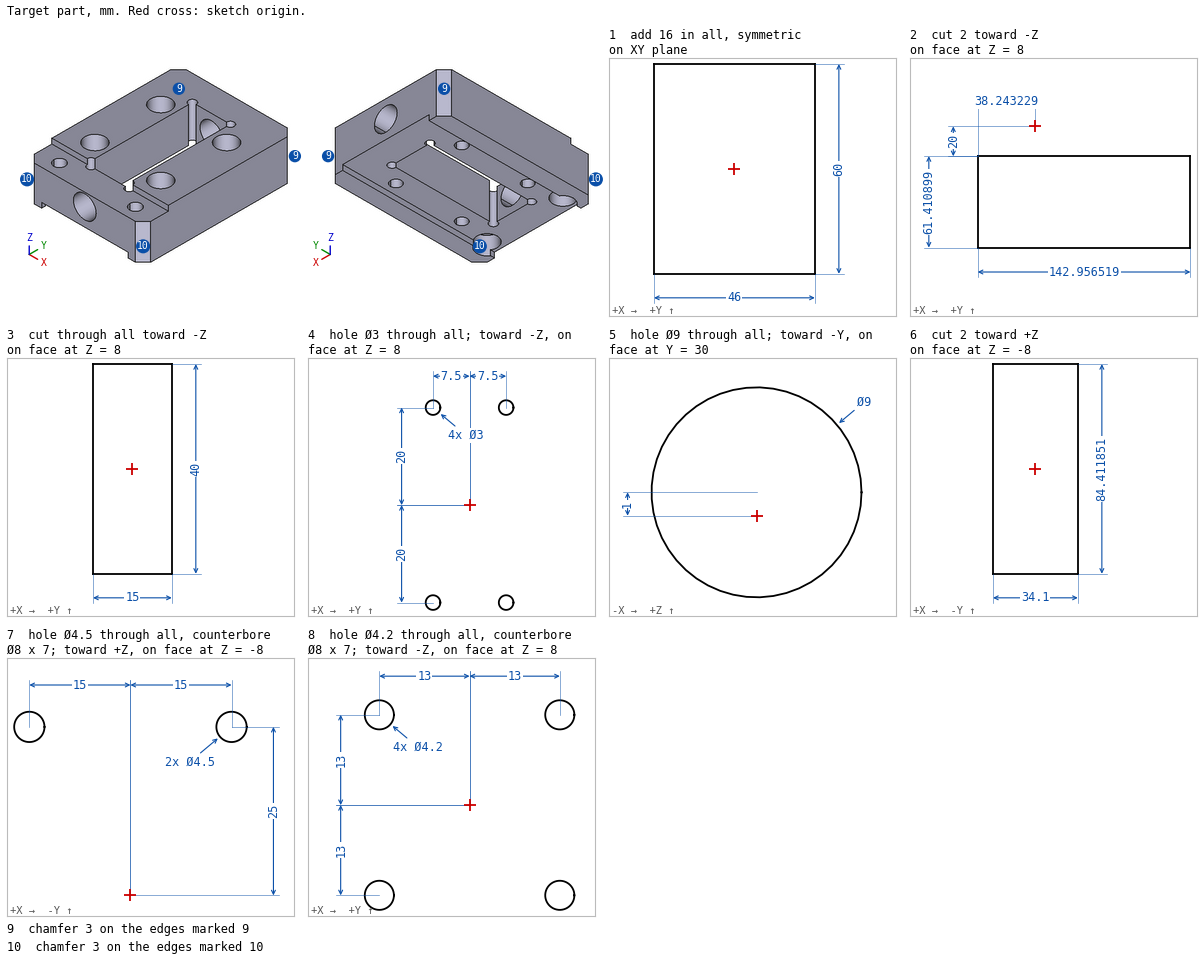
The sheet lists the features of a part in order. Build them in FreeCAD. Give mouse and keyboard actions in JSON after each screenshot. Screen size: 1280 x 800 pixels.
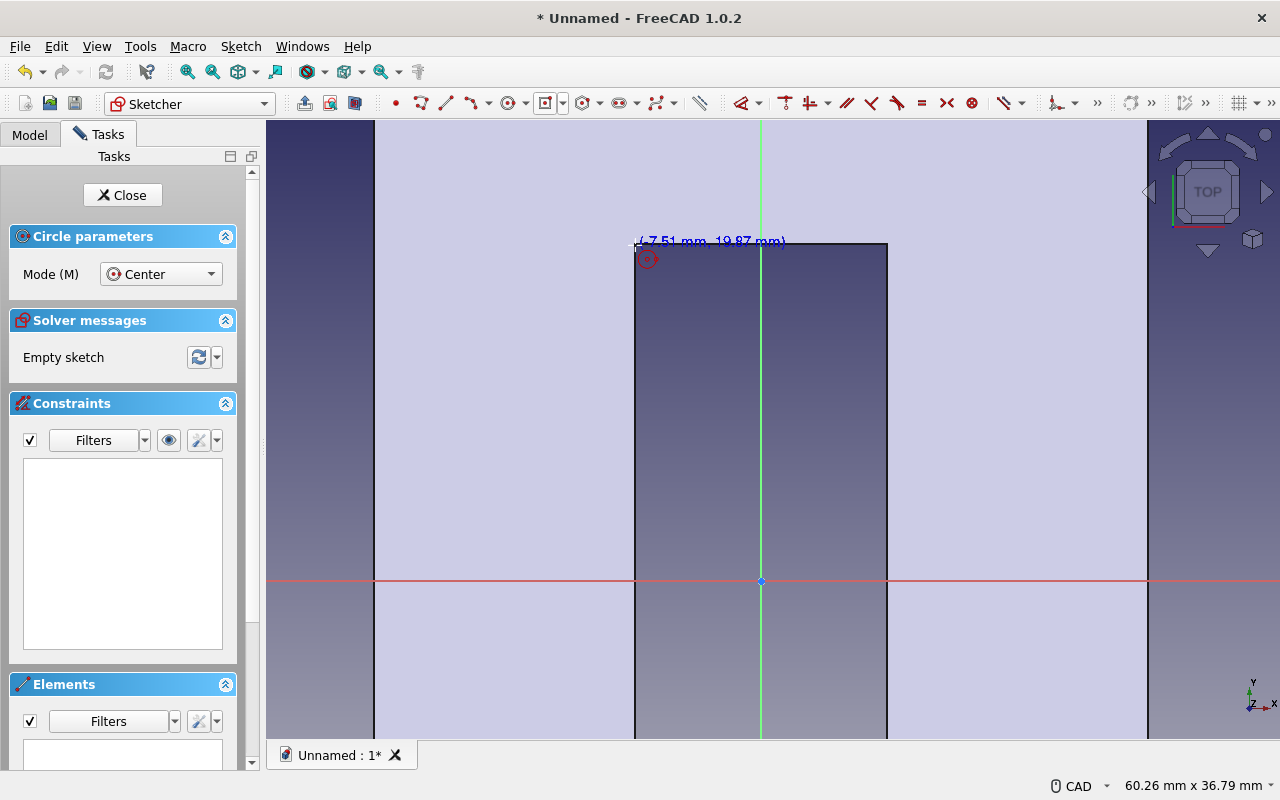
{"action": "left_click", "coordinate": [635, 244]}
{"action": "left_click", "coordinate": [653, 227]}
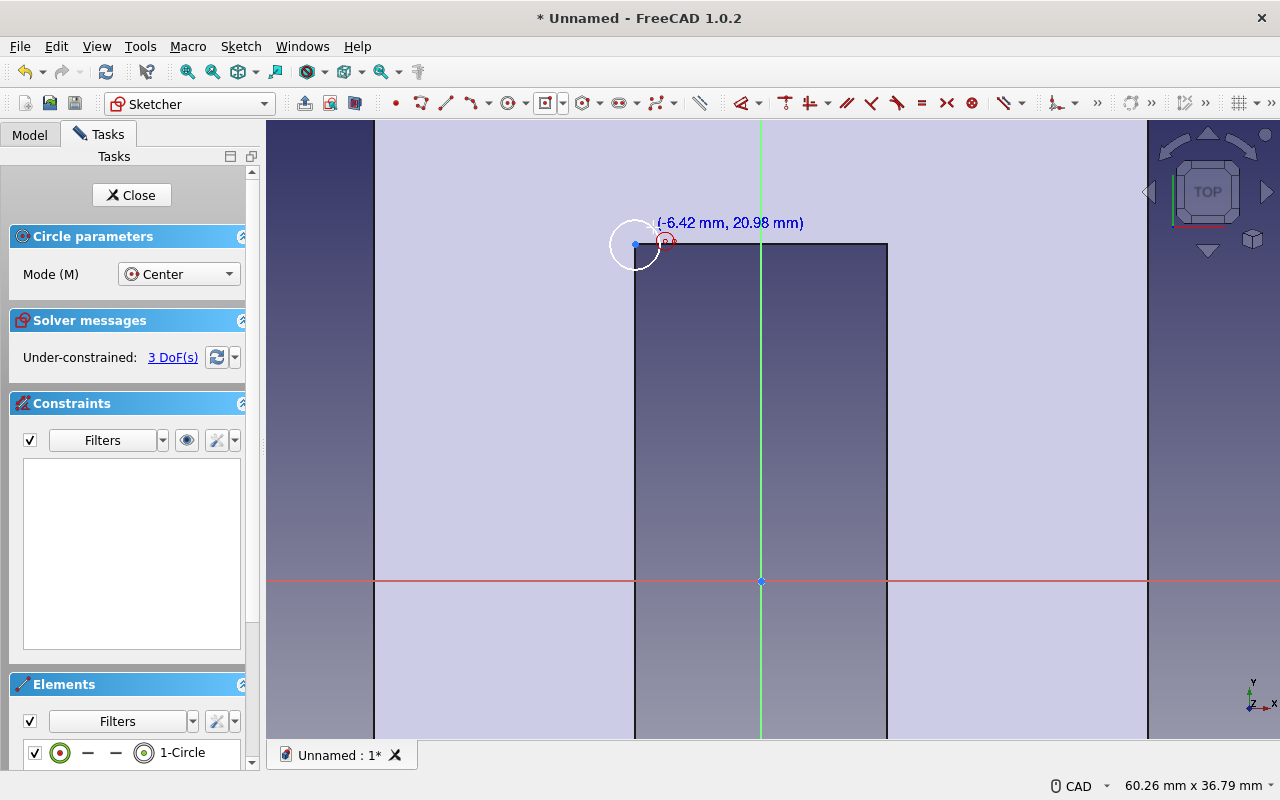
{"action": "left_click", "coordinate": [887, 244]}
{"action": "left_click", "coordinate": [905, 227]}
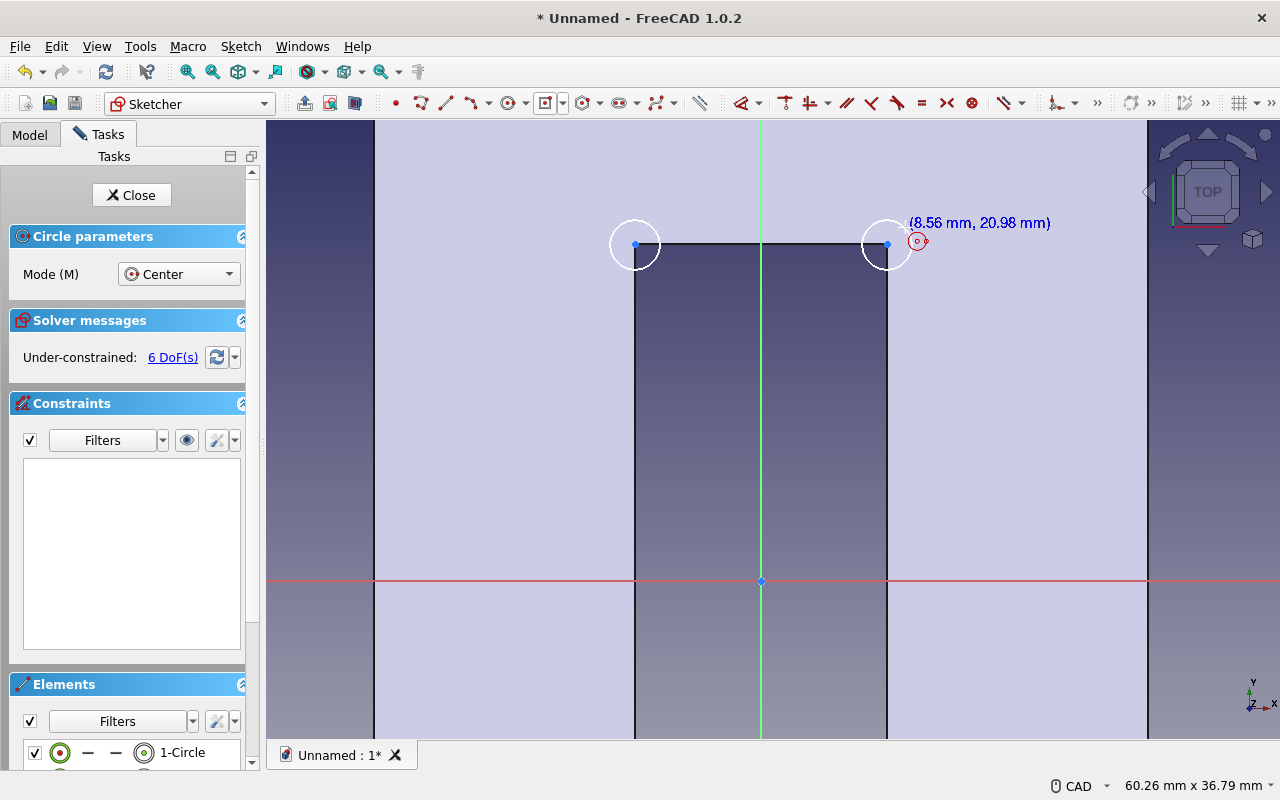
{"action": "scroll", "coordinate": [636, 245], "scroll_direction": "down", "scroll_amount": 3}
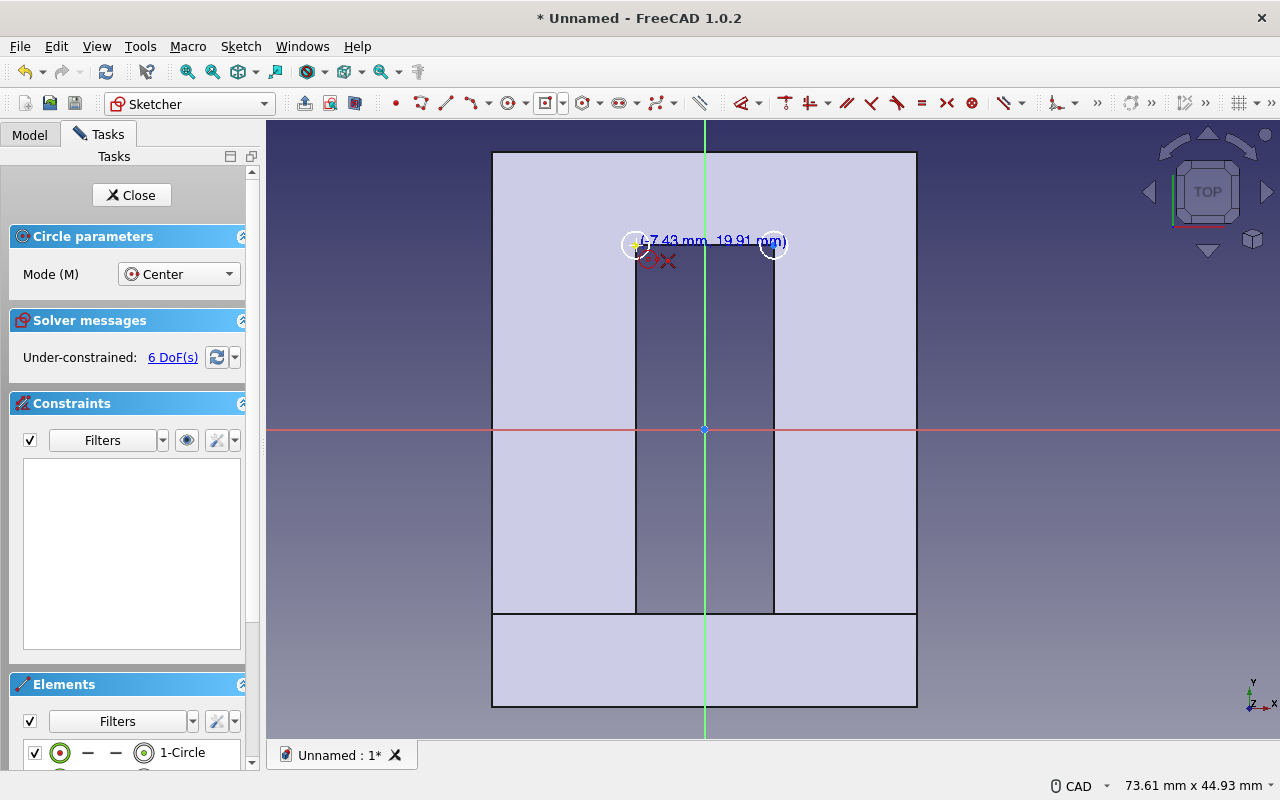
{"action": "scroll", "coordinate": [636, 614], "scroll_direction": "up", "scroll_amount": 3}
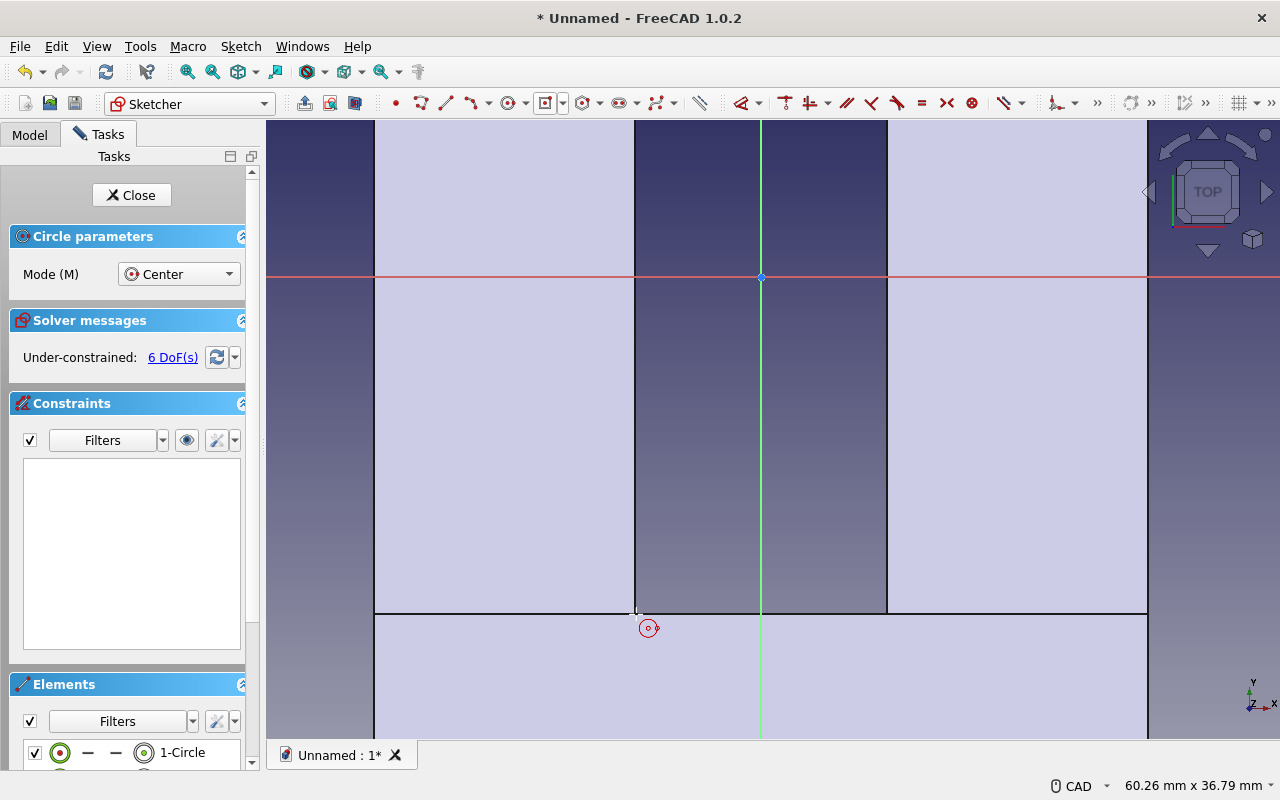
{"action": "left_click", "coordinate": [635, 614]}
{"action": "left_click", "coordinate": [653, 596]}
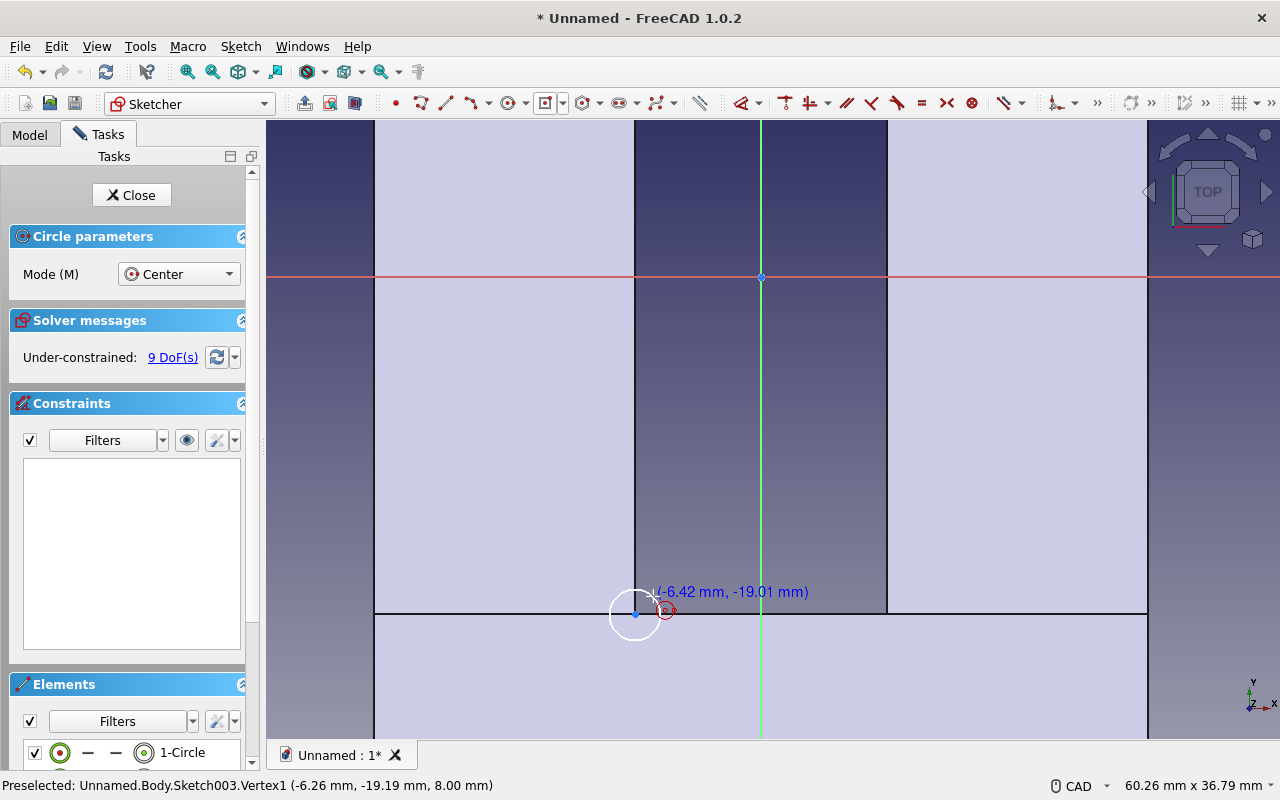
{"action": "left_click", "coordinate": [887, 614]}
{"action": "left_click", "coordinate": [905, 596]}
{"action": "key", "text": "Escape"}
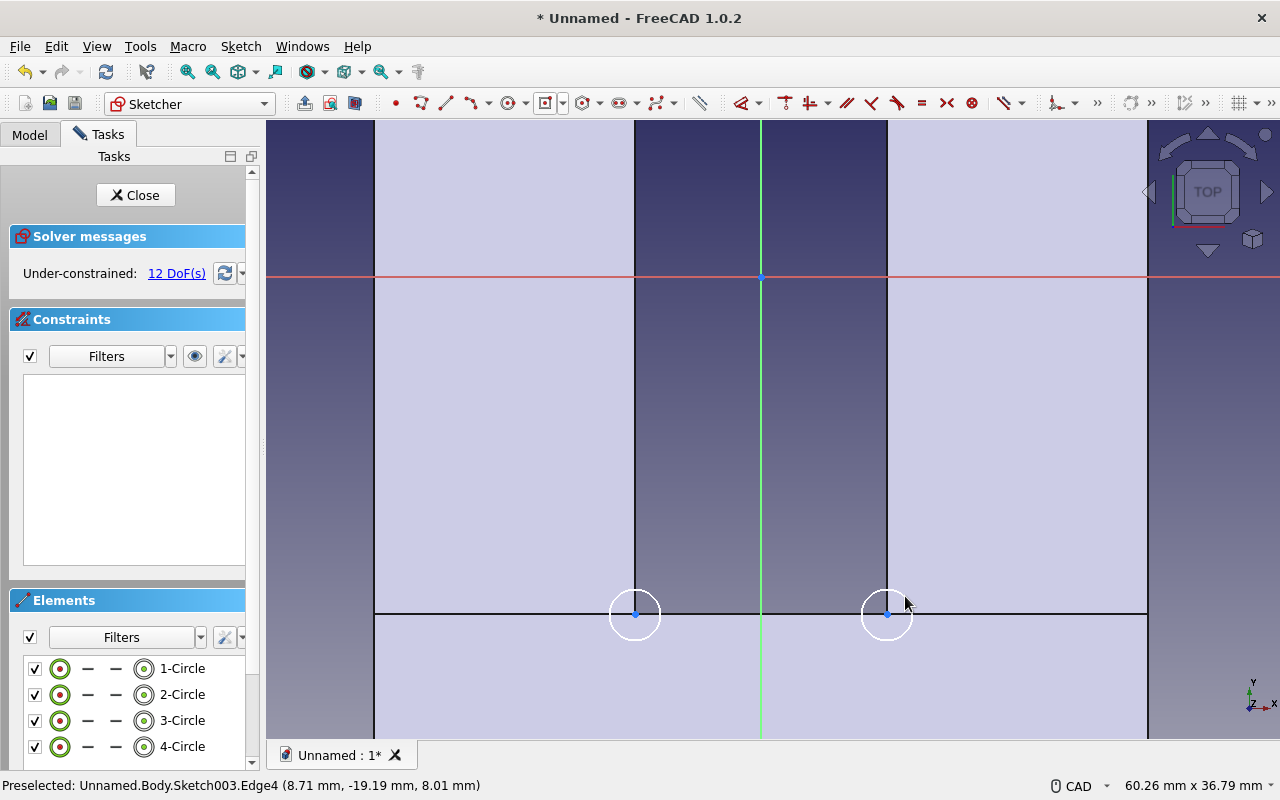
{"action": "scroll", "coordinate": [636, 615], "scroll_direction": "down", "scroll_amount": 3}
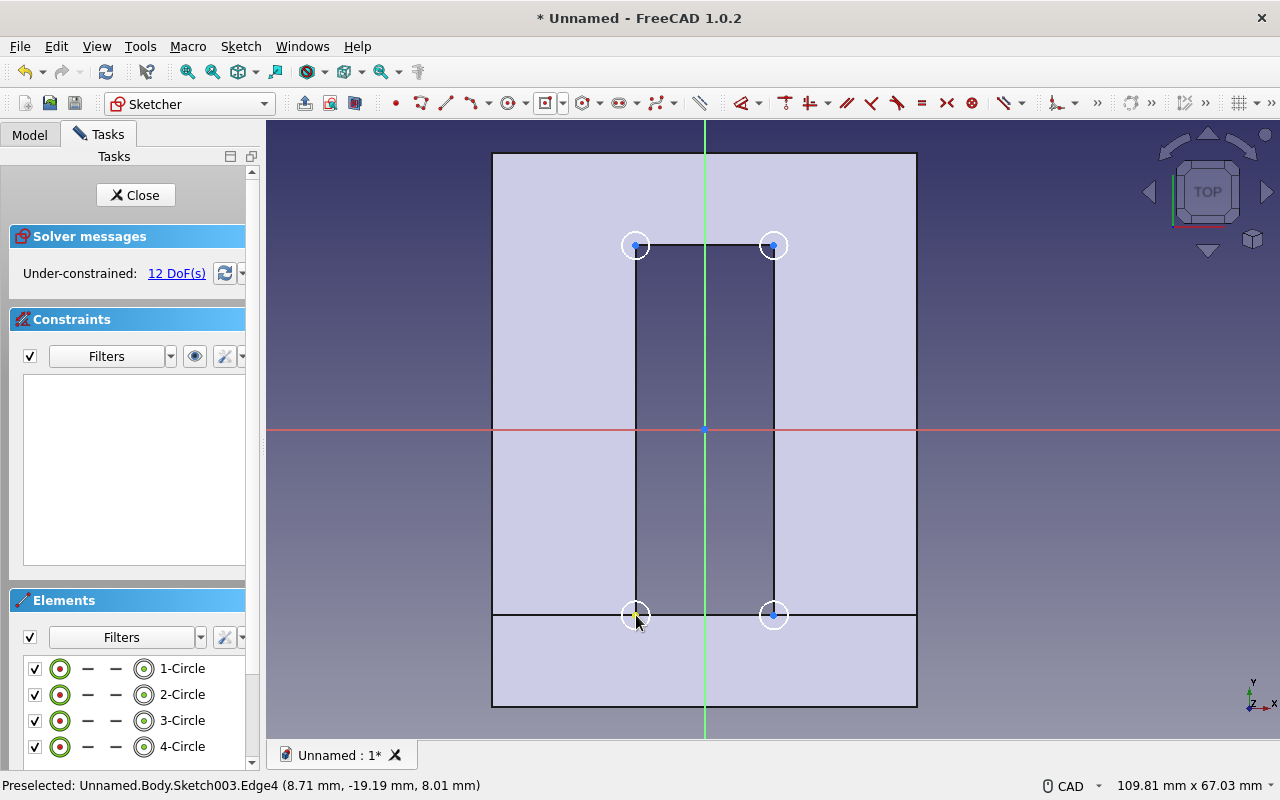
{"action": "left_click", "coordinate": [645, 236]}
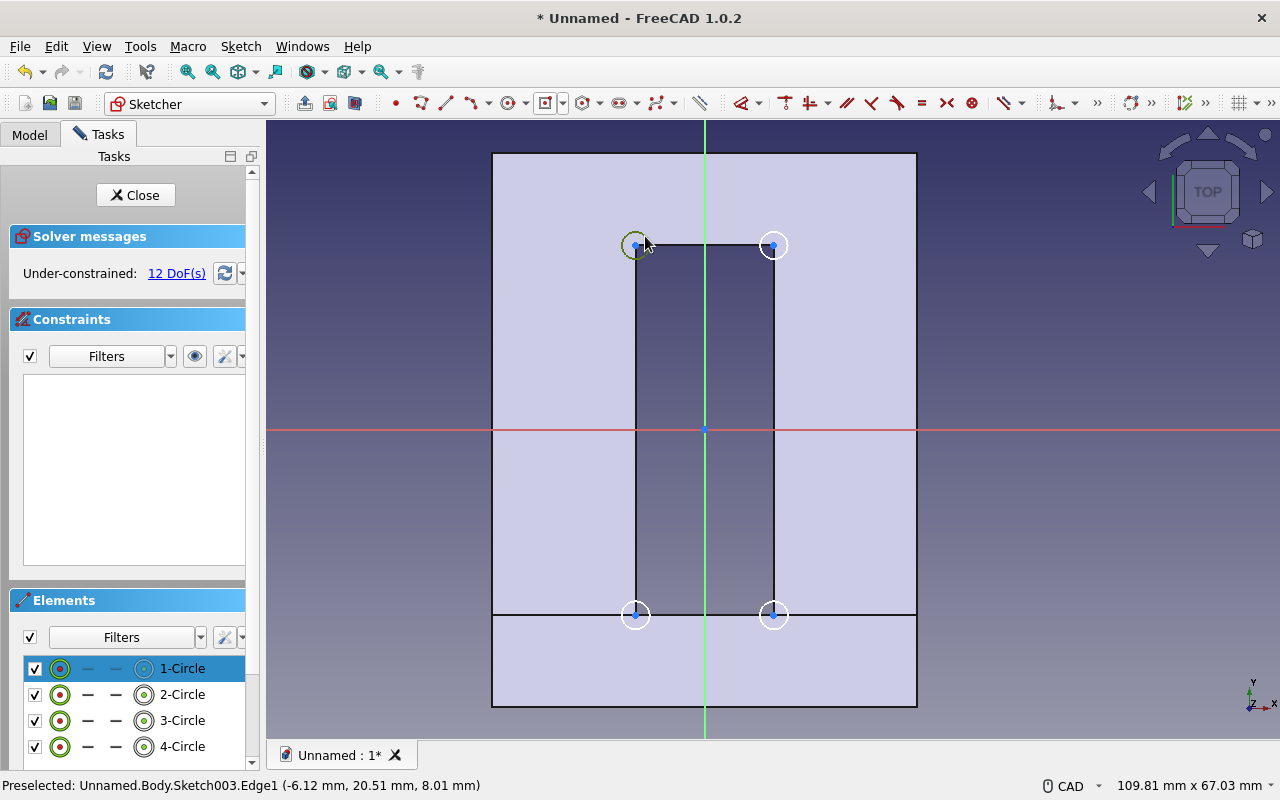
{"action": "left_click", "coordinate": [783, 236]}